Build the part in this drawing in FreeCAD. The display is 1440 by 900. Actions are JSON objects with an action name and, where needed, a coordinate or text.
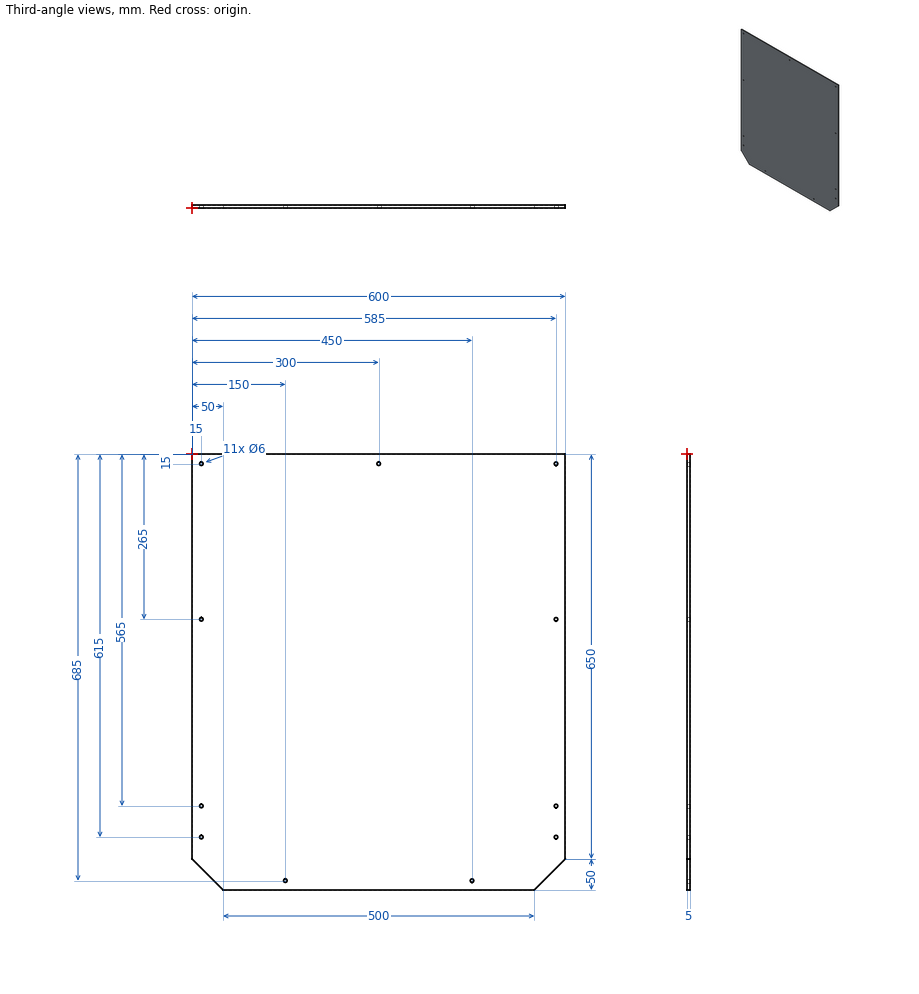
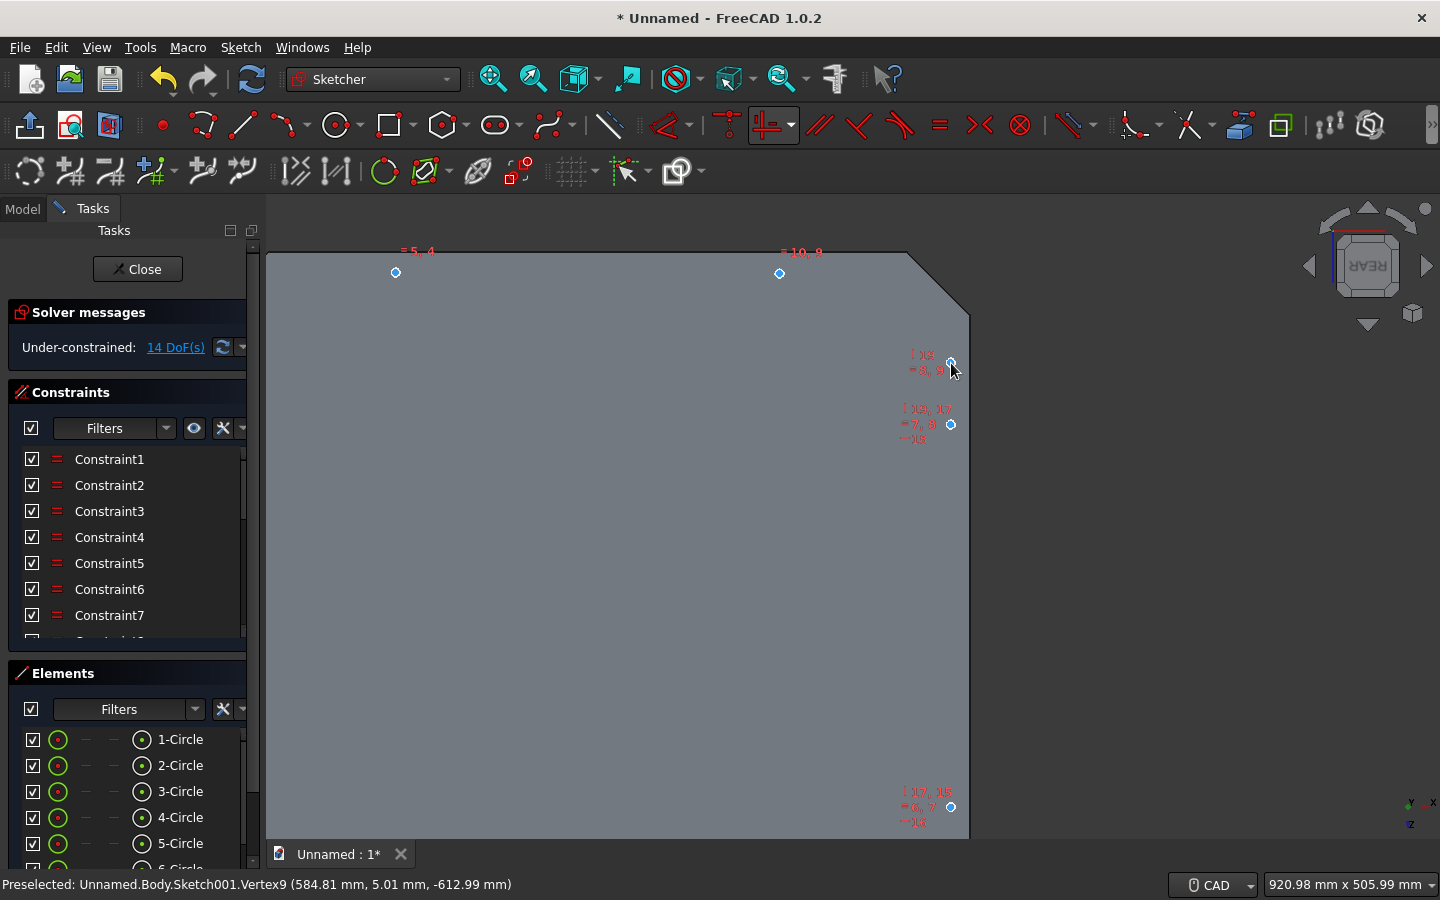
{"action": "scroll", "coordinate": [951, 362], "scroll_direction": "down", "scroll_amount": 4}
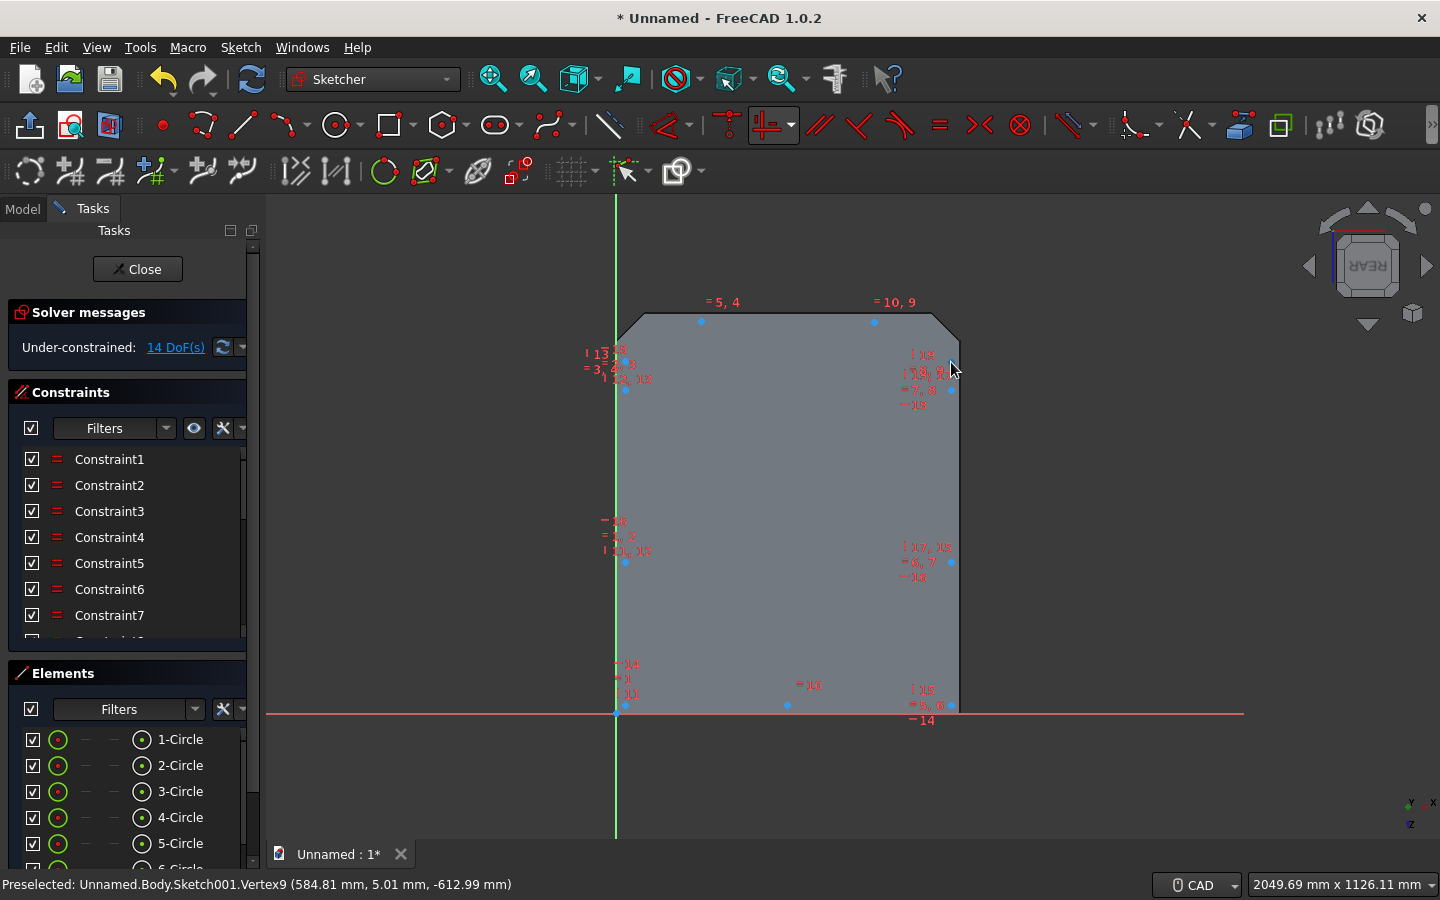
{"action": "left_click", "coordinate": [625, 362]}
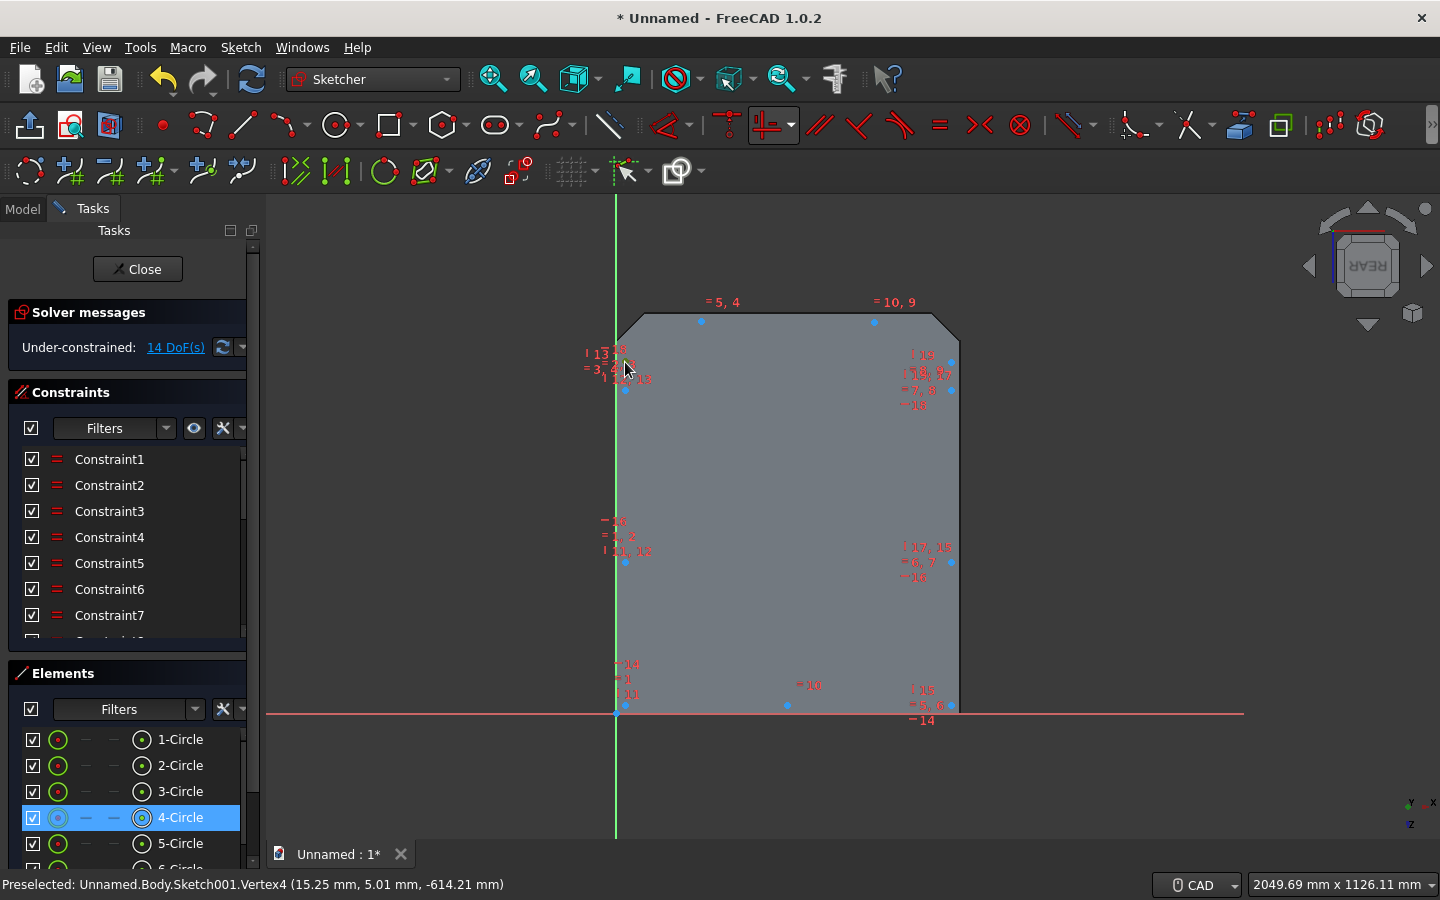
{"action": "left_click", "coordinate": [951, 362]}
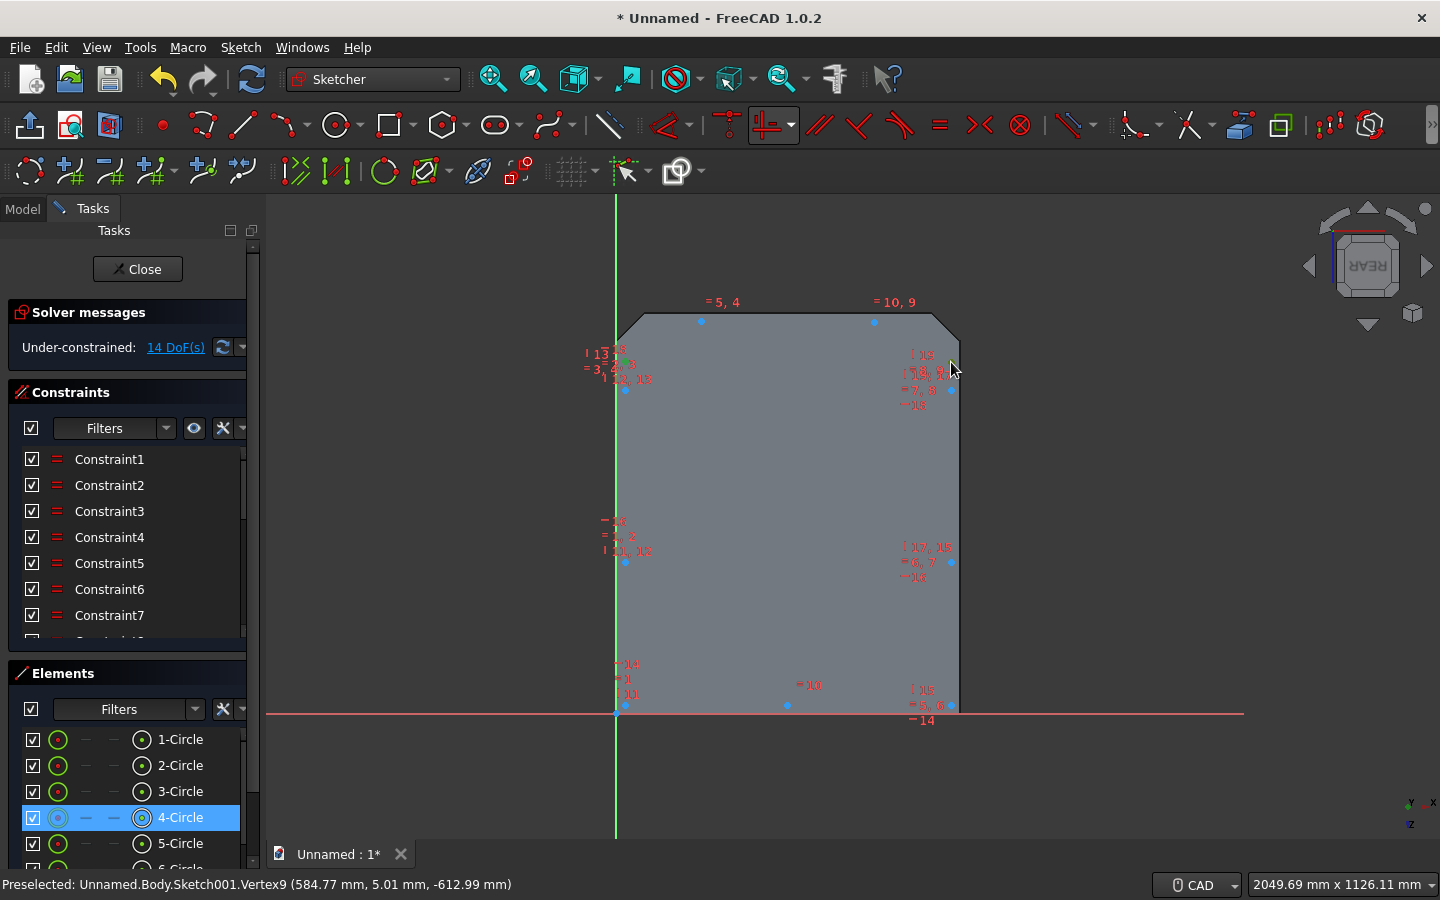
{"action": "key", "text": "h"}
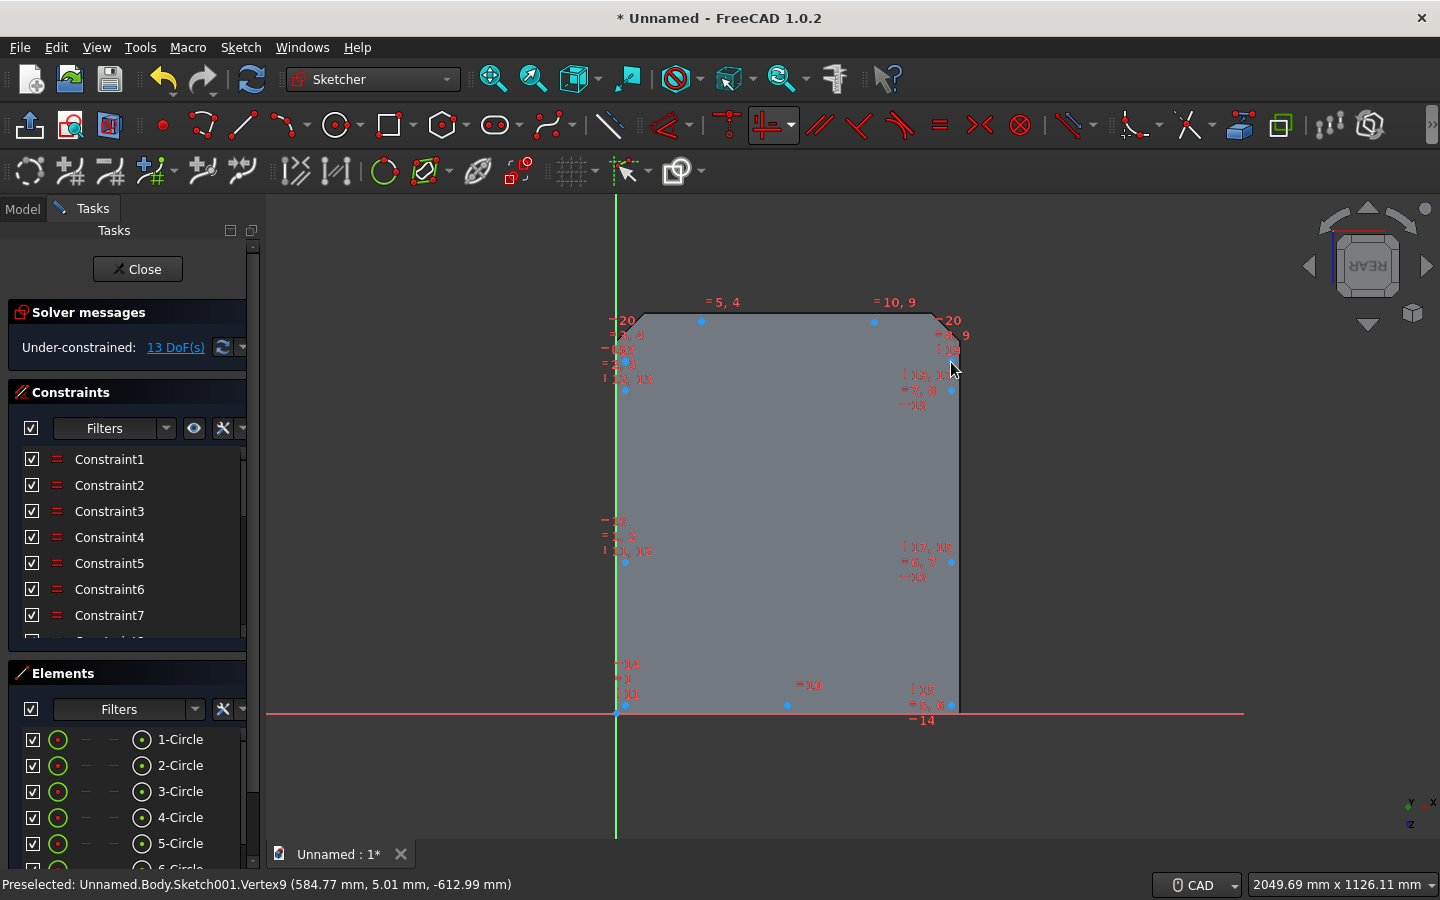
{"action": "left_click", "coordinate": [702, 322]}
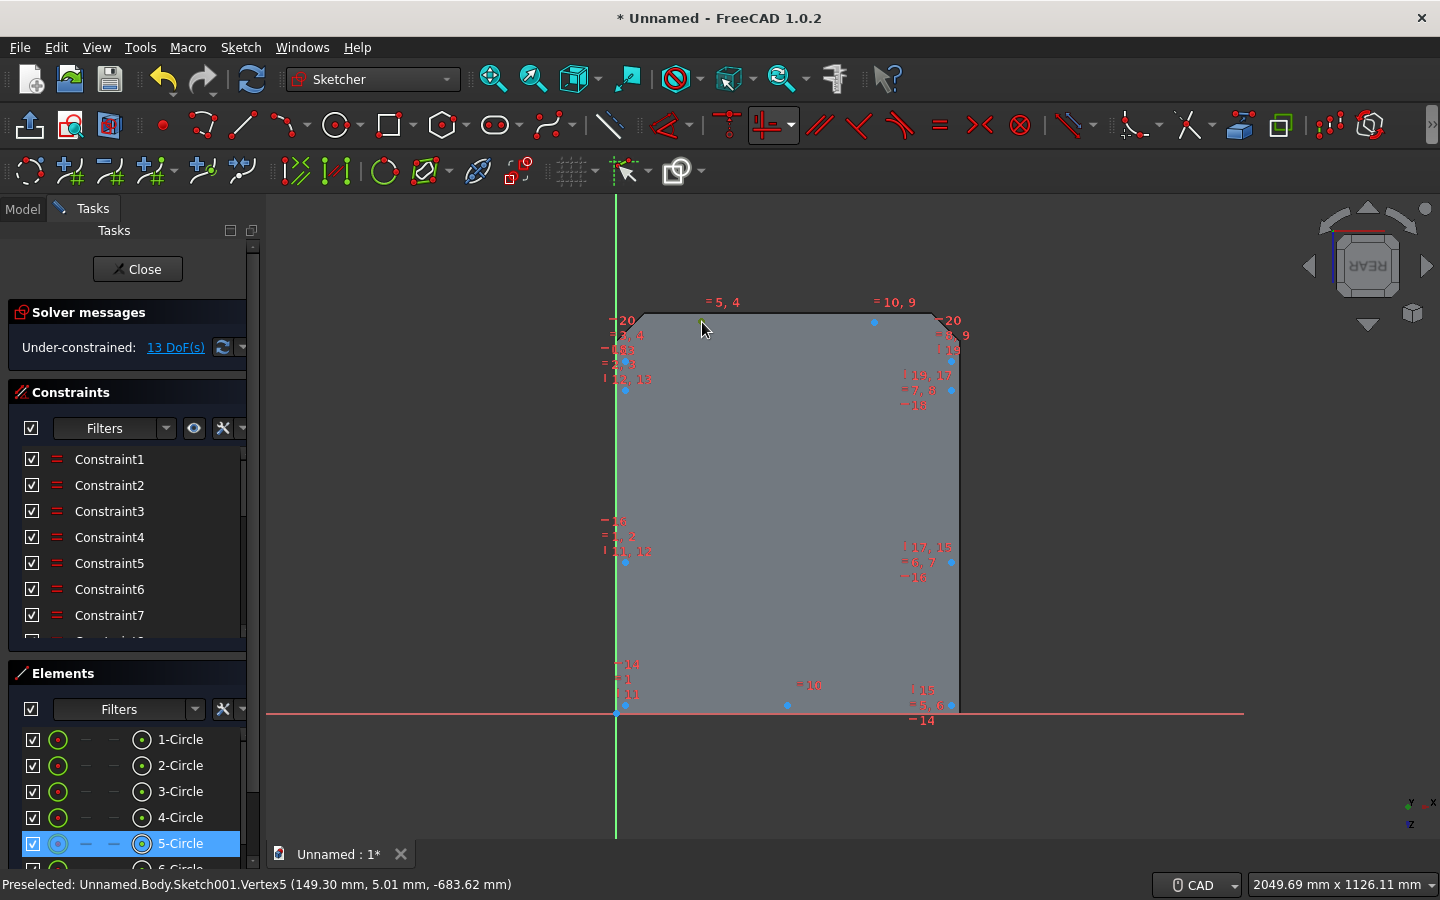
{"action": "left_click", "coordinate": [874, 322]}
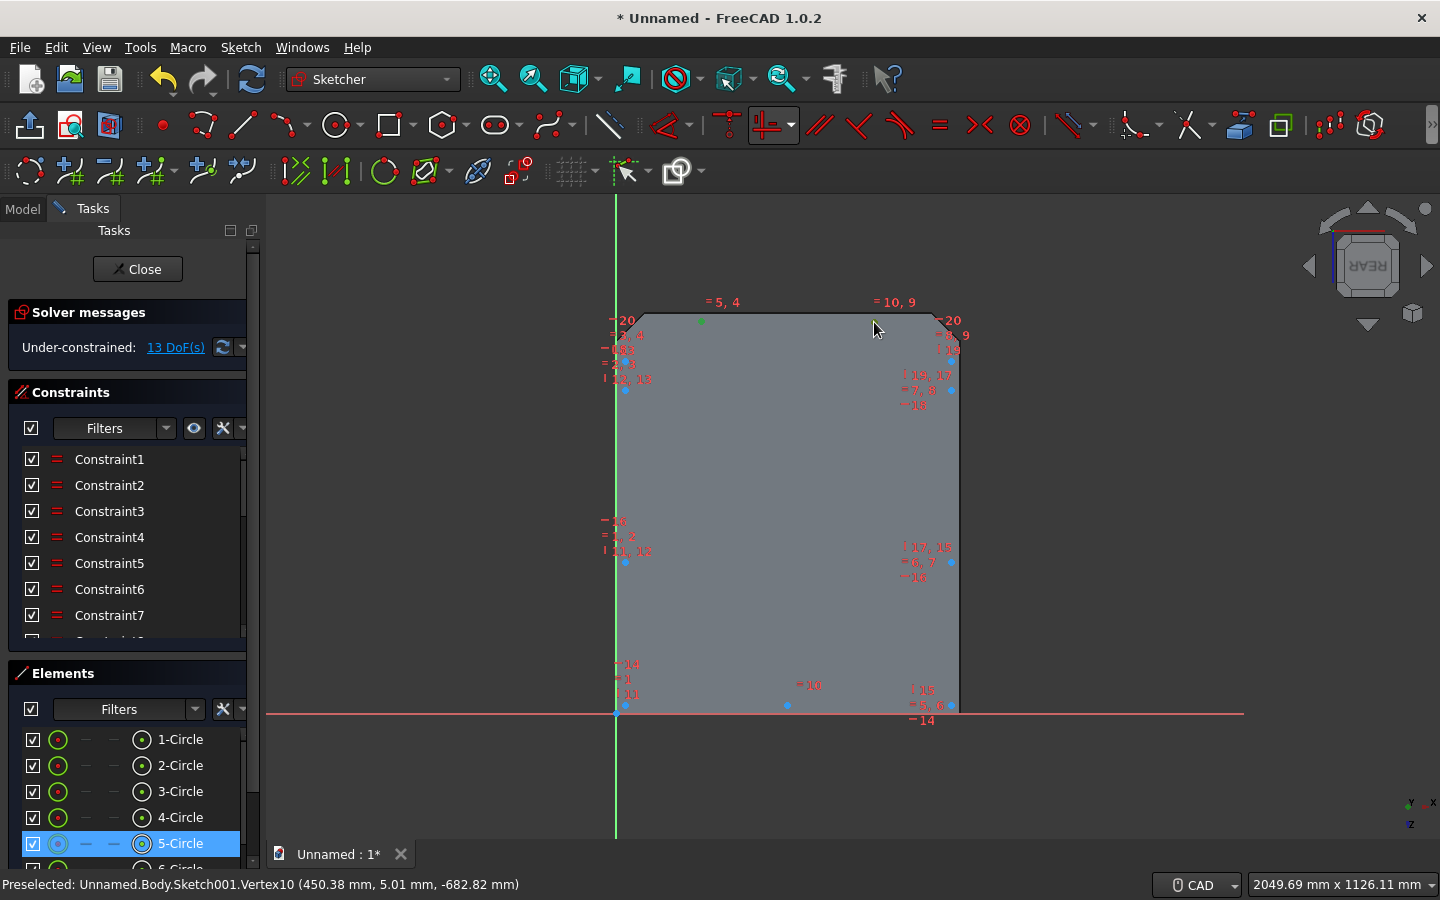
{"action": "key", "text": "h"}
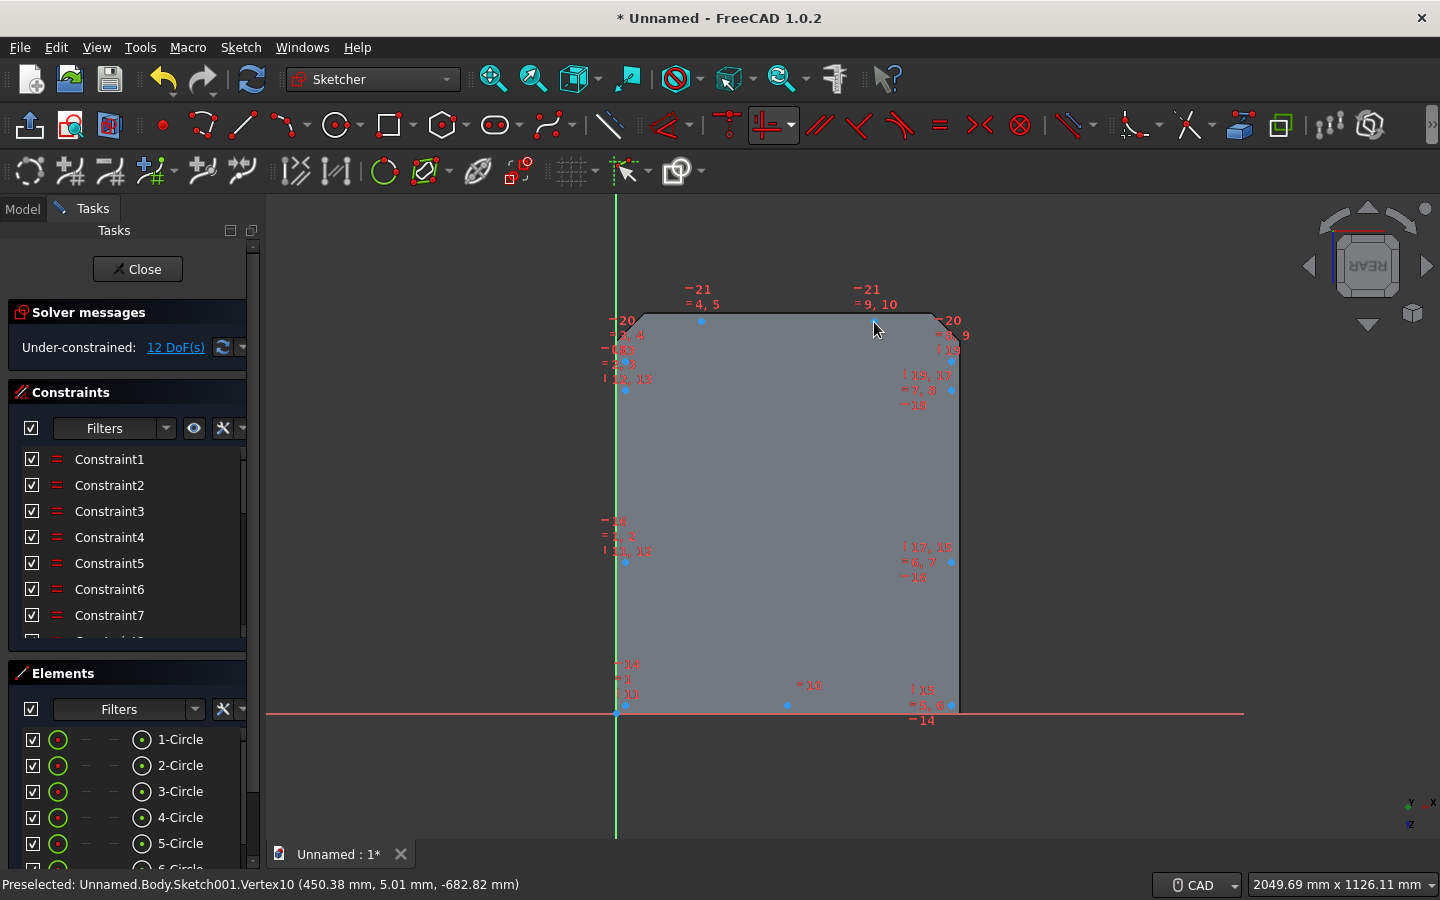
{"action": "left_click", "coordinate": [625, 705]}